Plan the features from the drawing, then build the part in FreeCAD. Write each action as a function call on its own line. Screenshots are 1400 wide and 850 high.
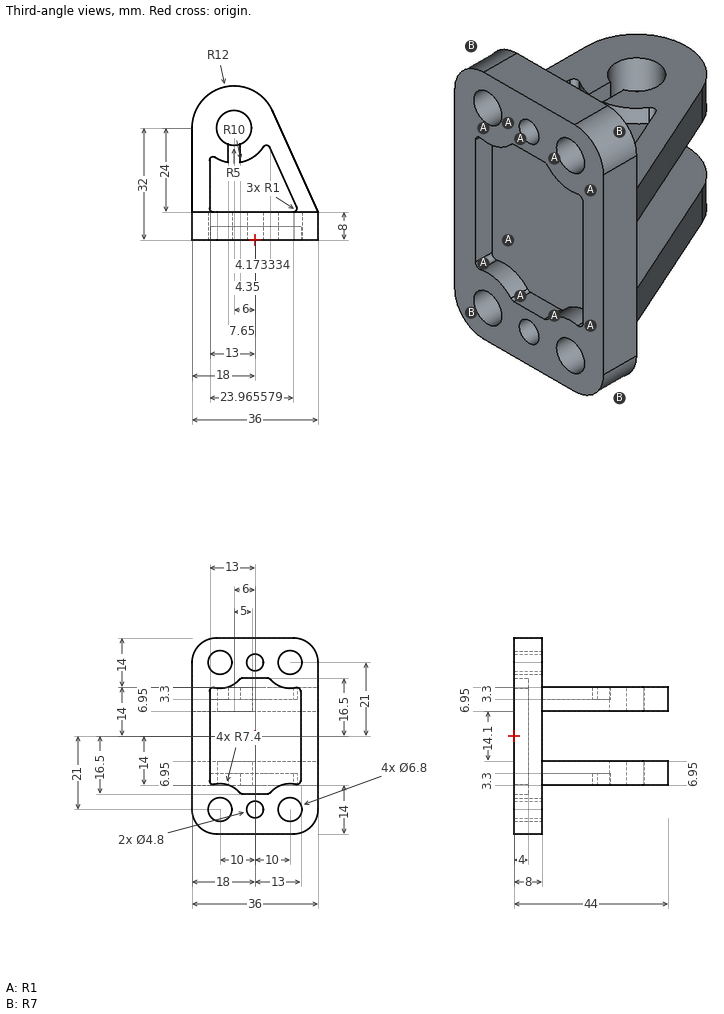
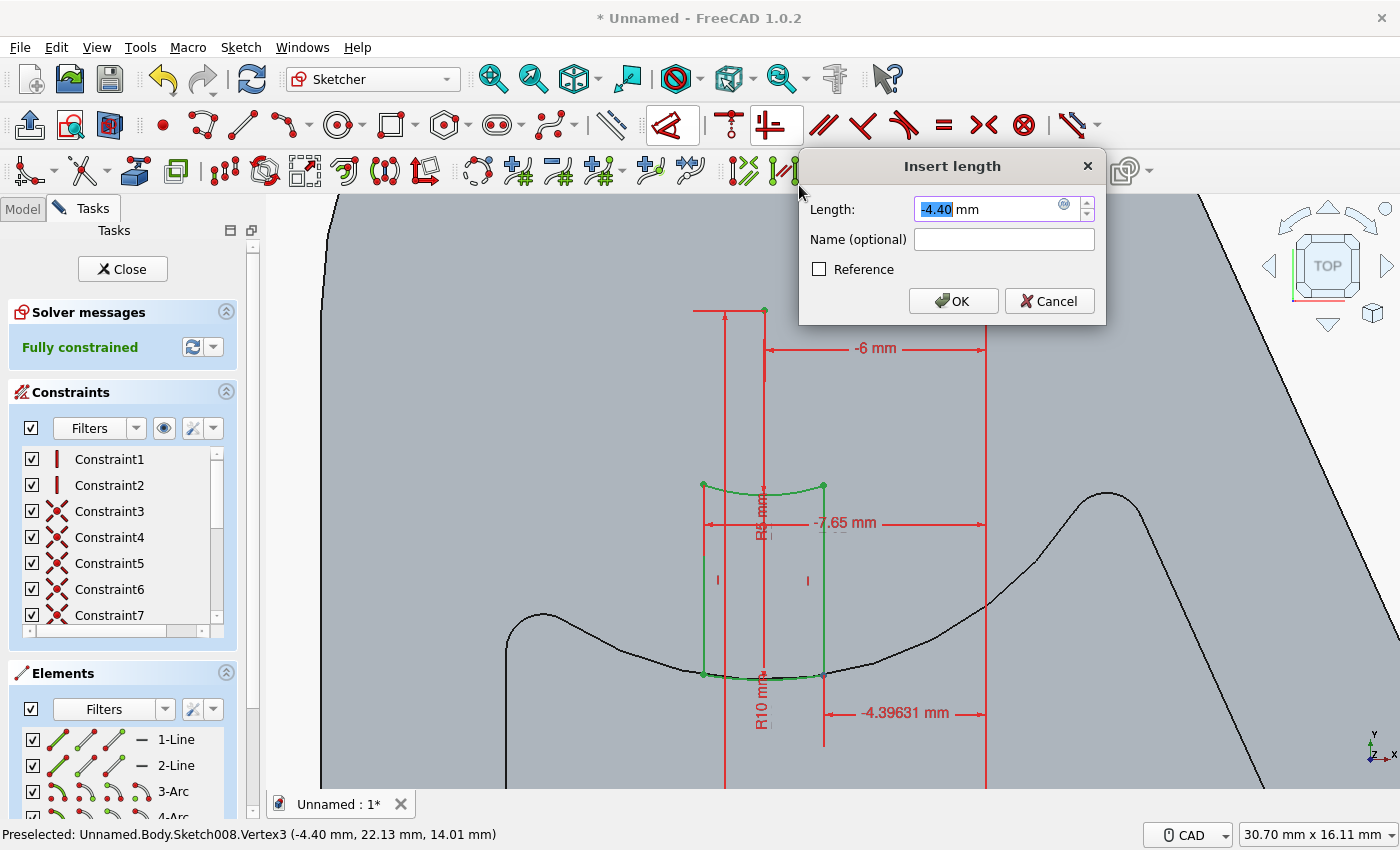
text(-4.35)
key(Return)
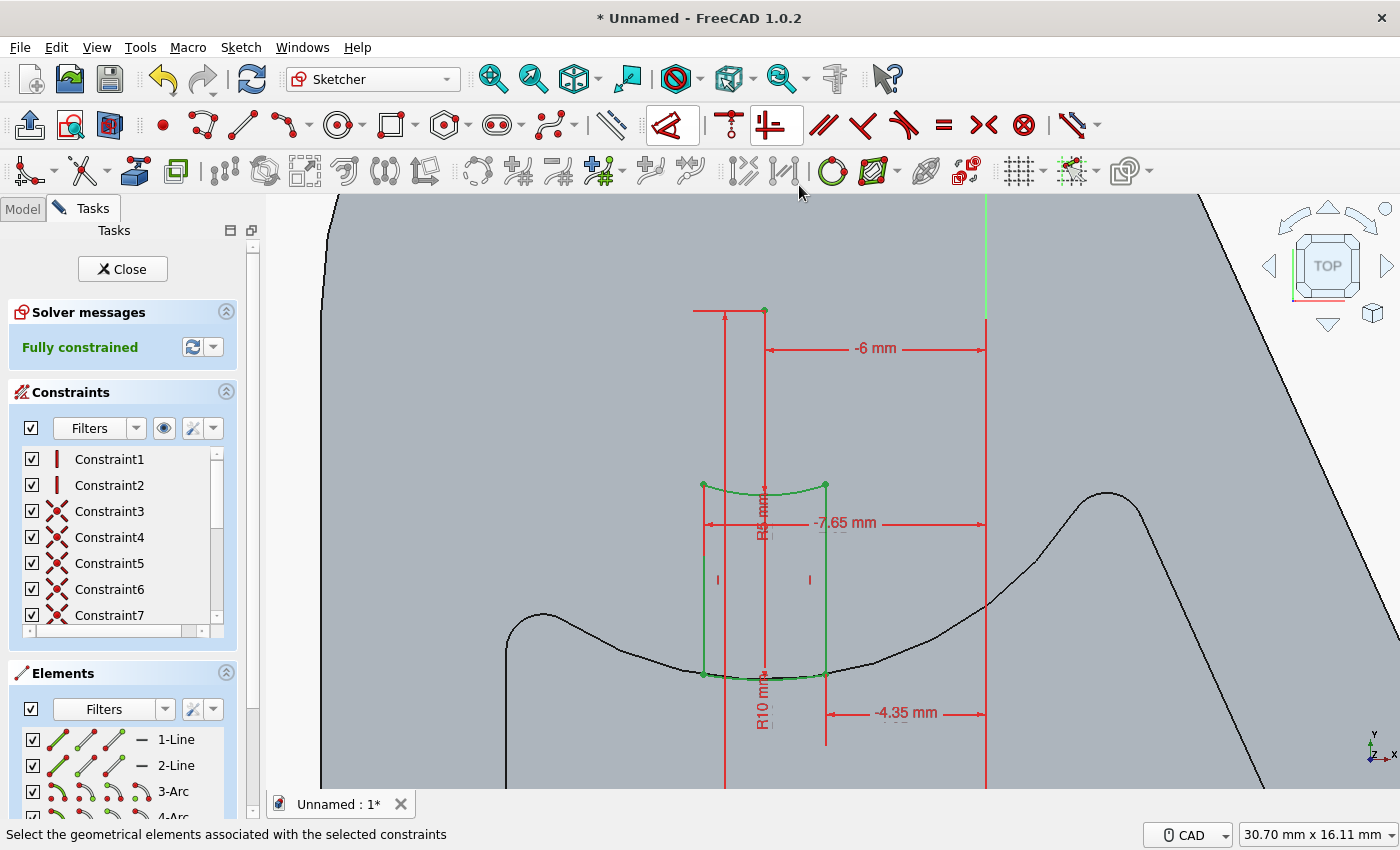
click(123, 269)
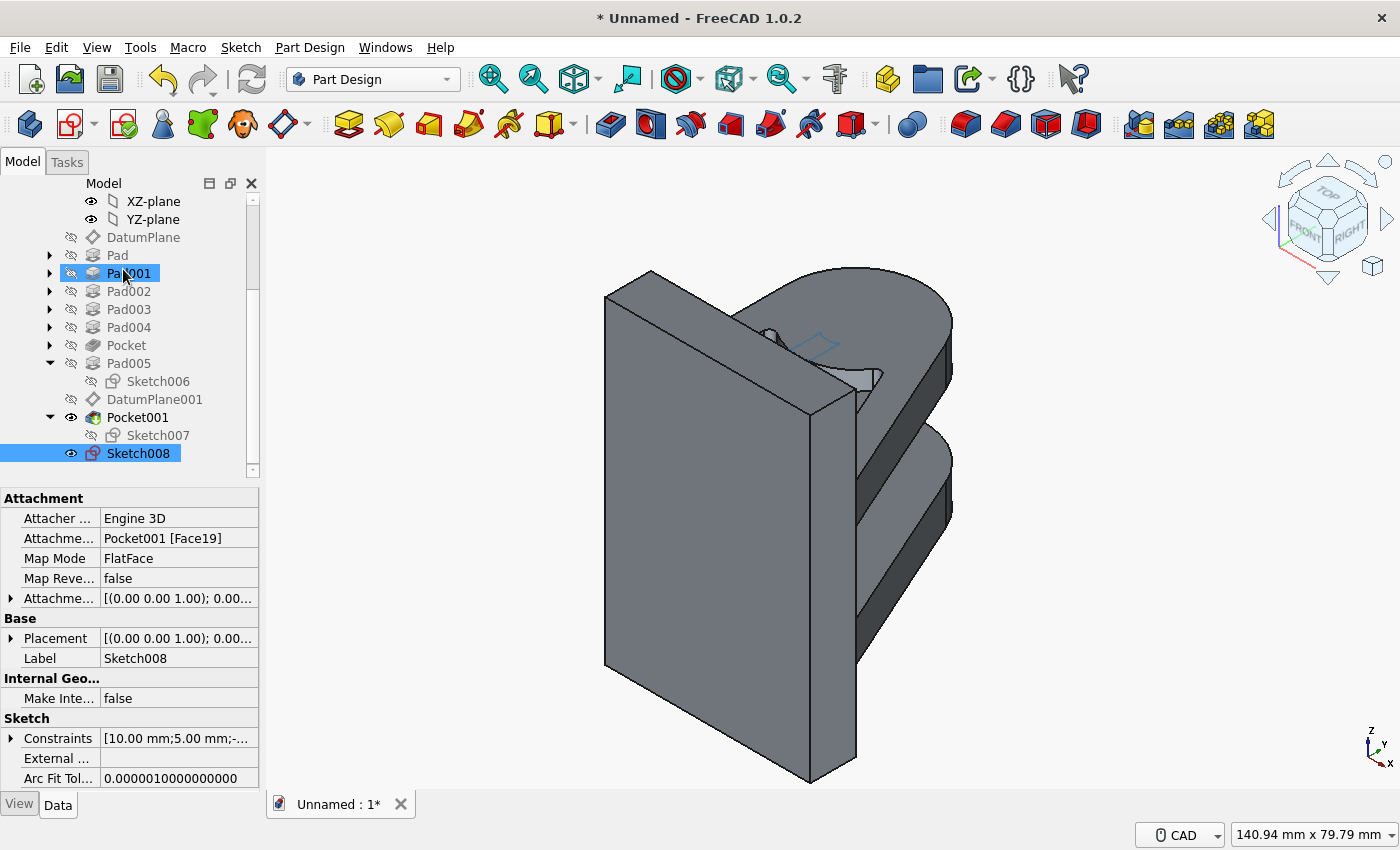
click(612, 124)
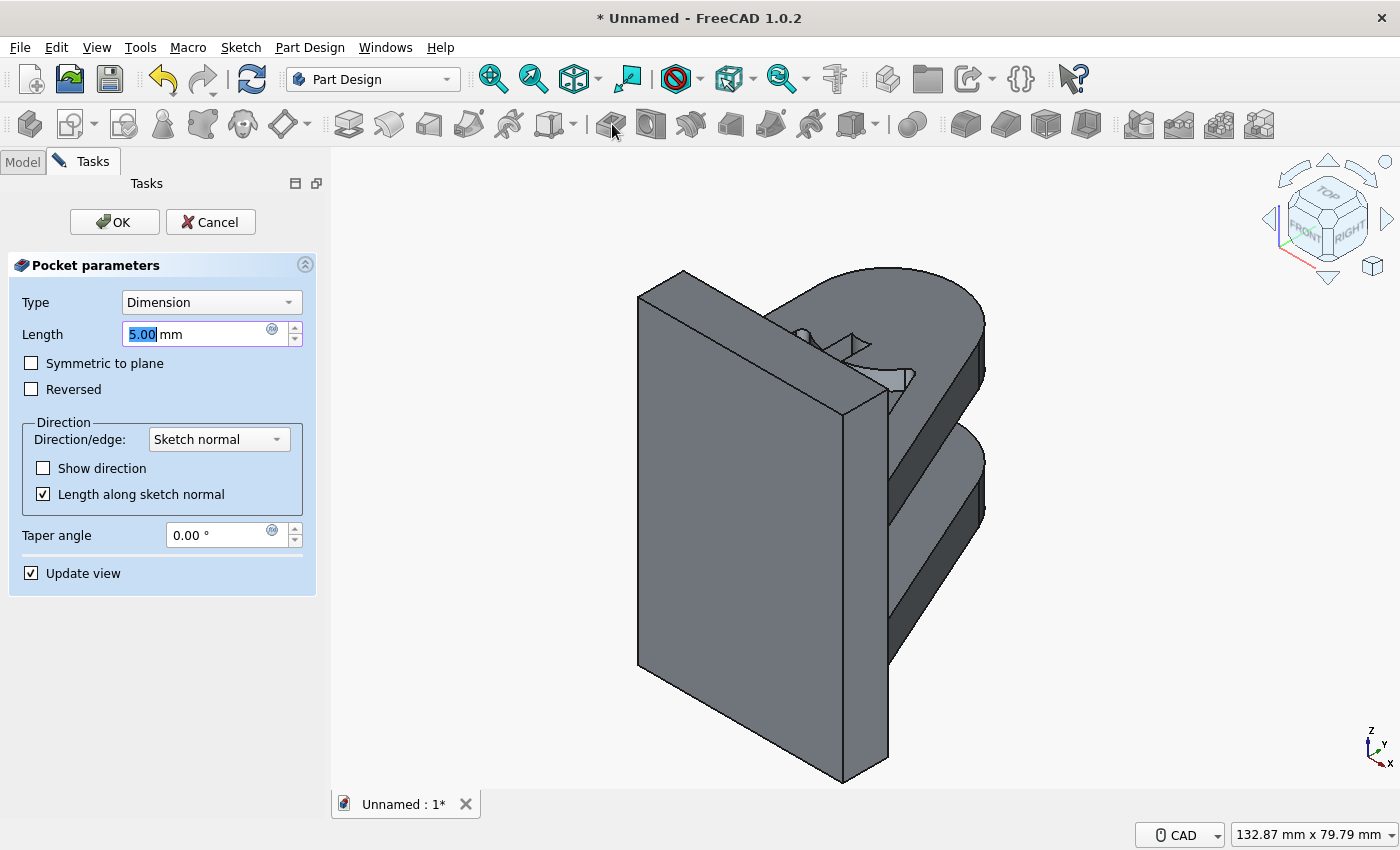
text(3.3)
key(Tab)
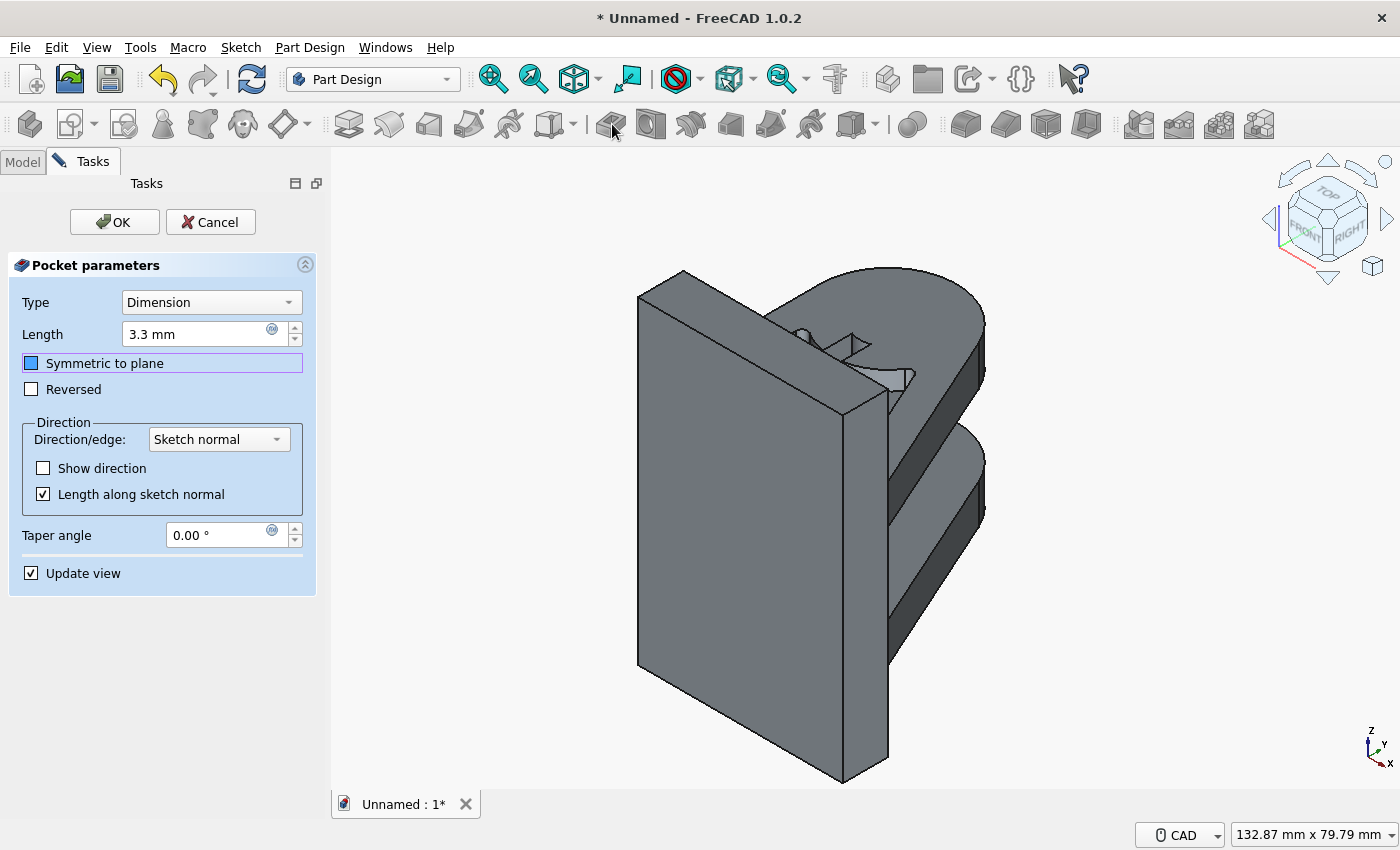
click(115, 222)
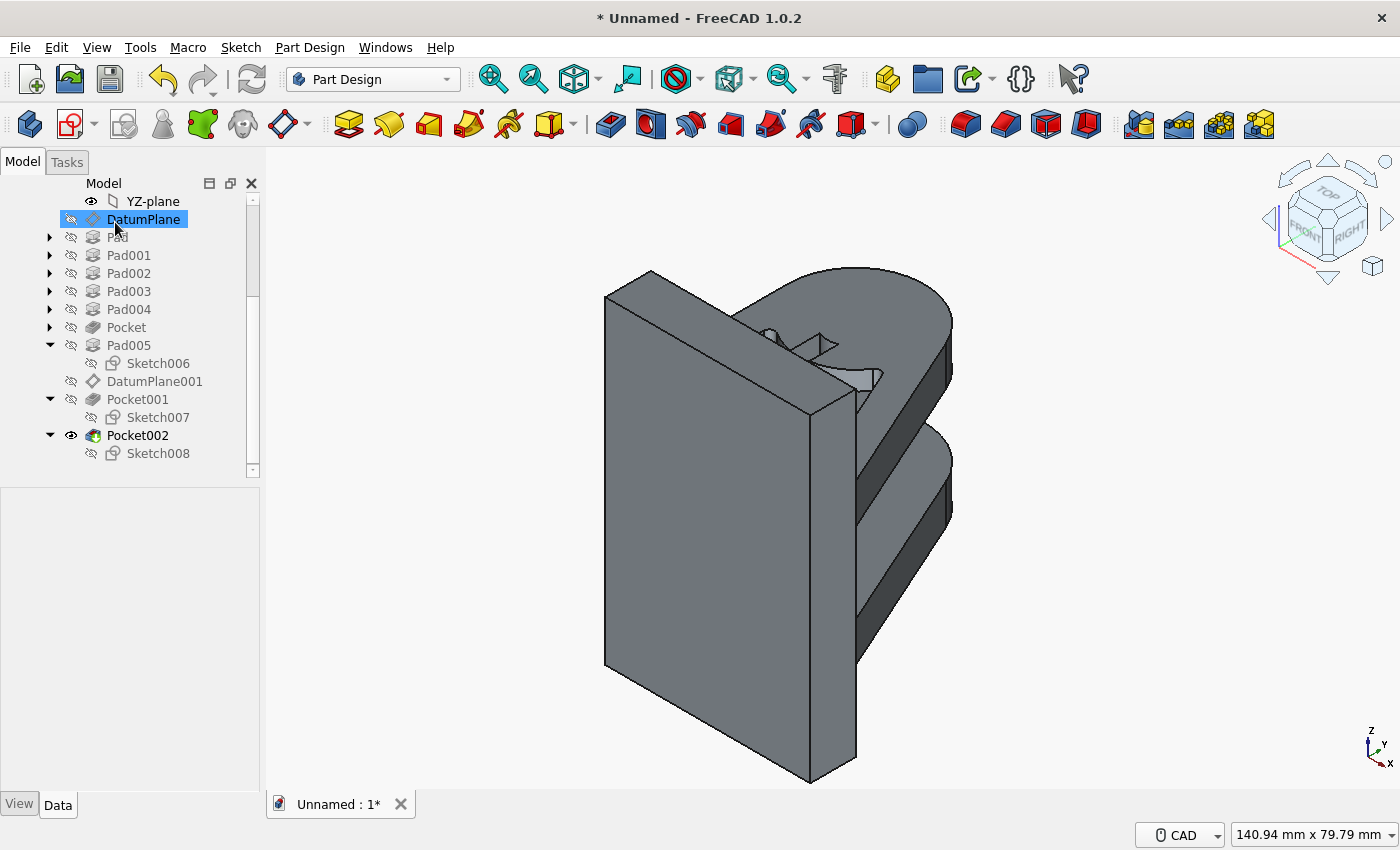
key(5)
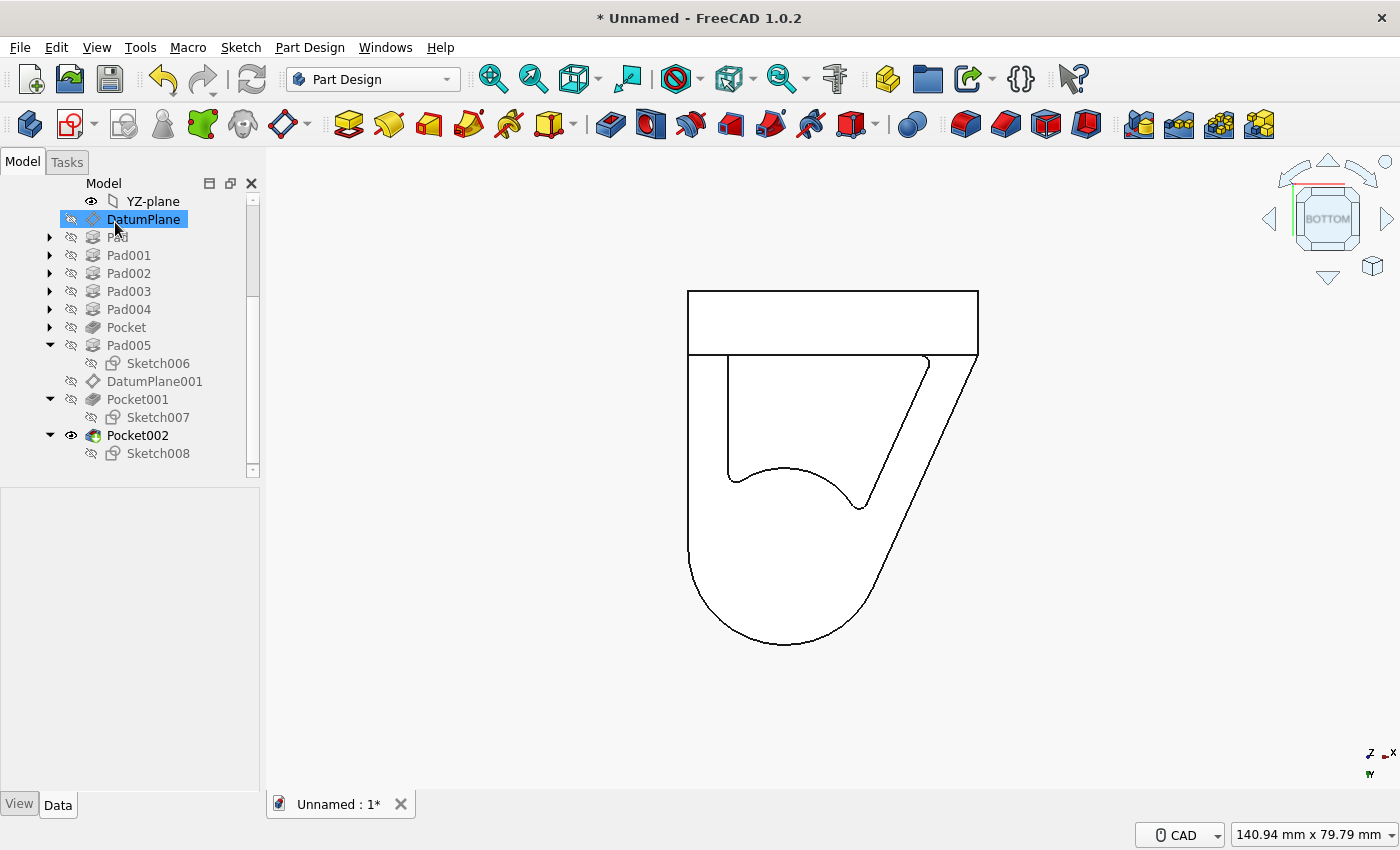
click(829, 409)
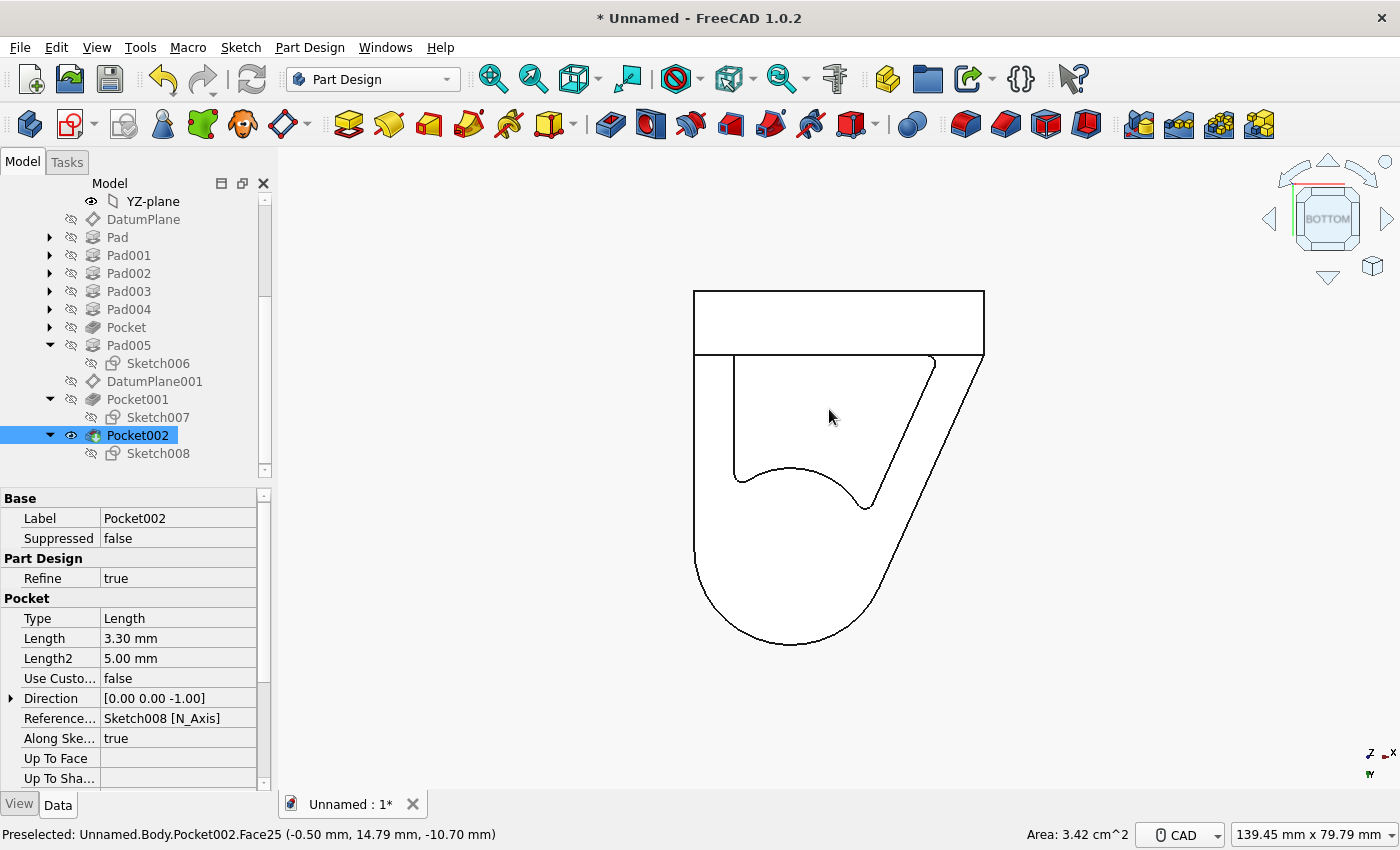
click(70, 124)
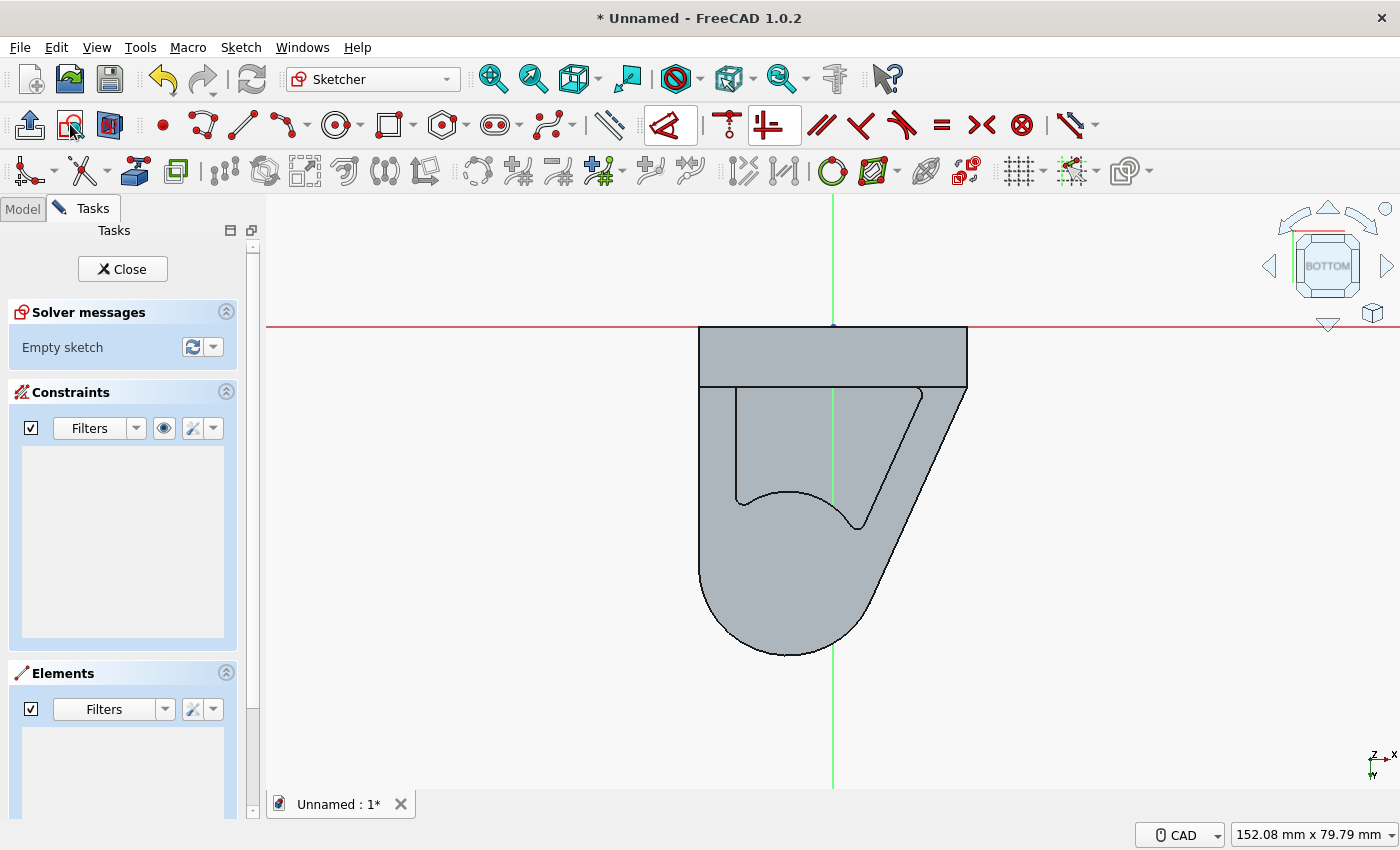
scroll(791, 514, up, 11)